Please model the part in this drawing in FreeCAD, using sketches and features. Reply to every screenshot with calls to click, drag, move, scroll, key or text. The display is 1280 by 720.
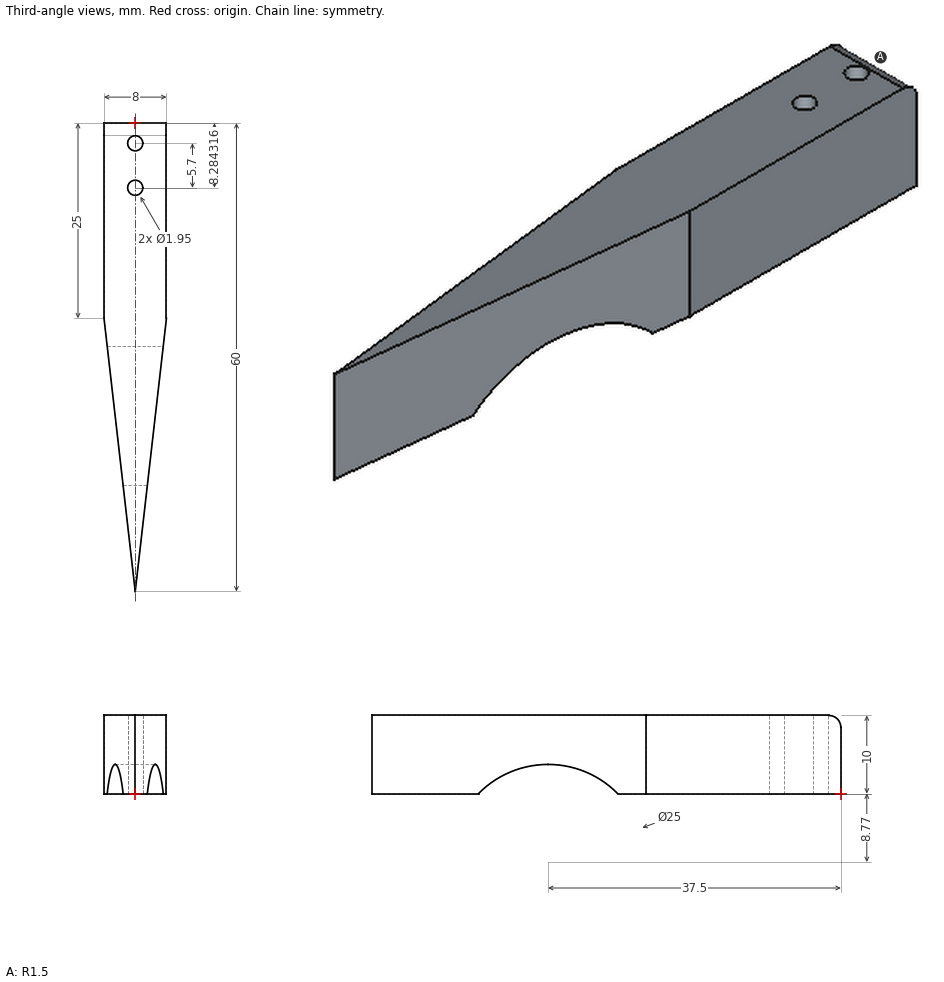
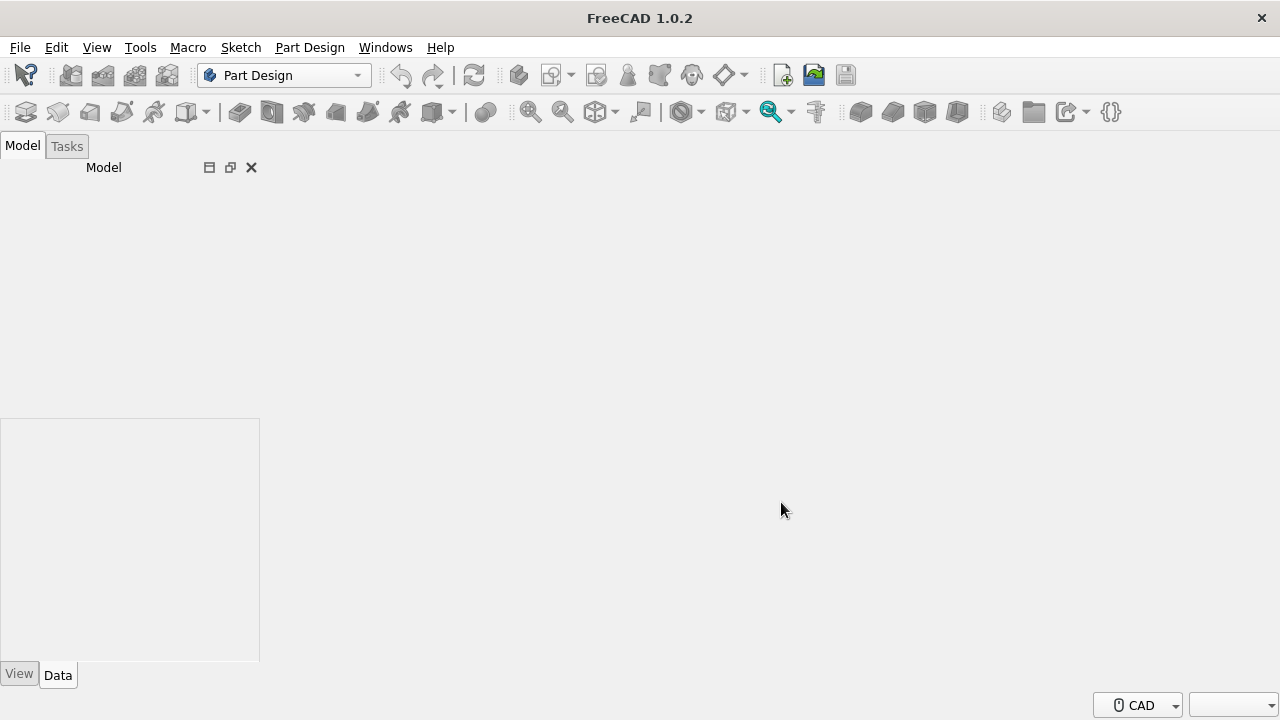
key(ctrl+n)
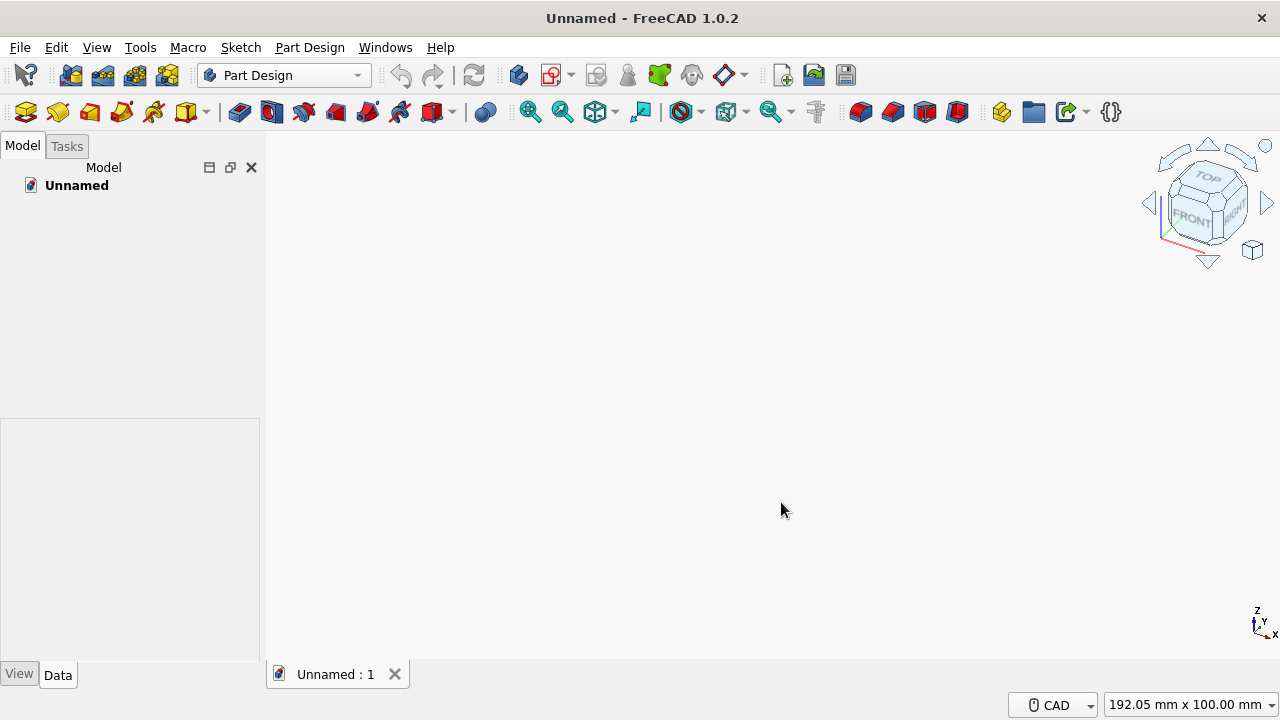
click(552, 76)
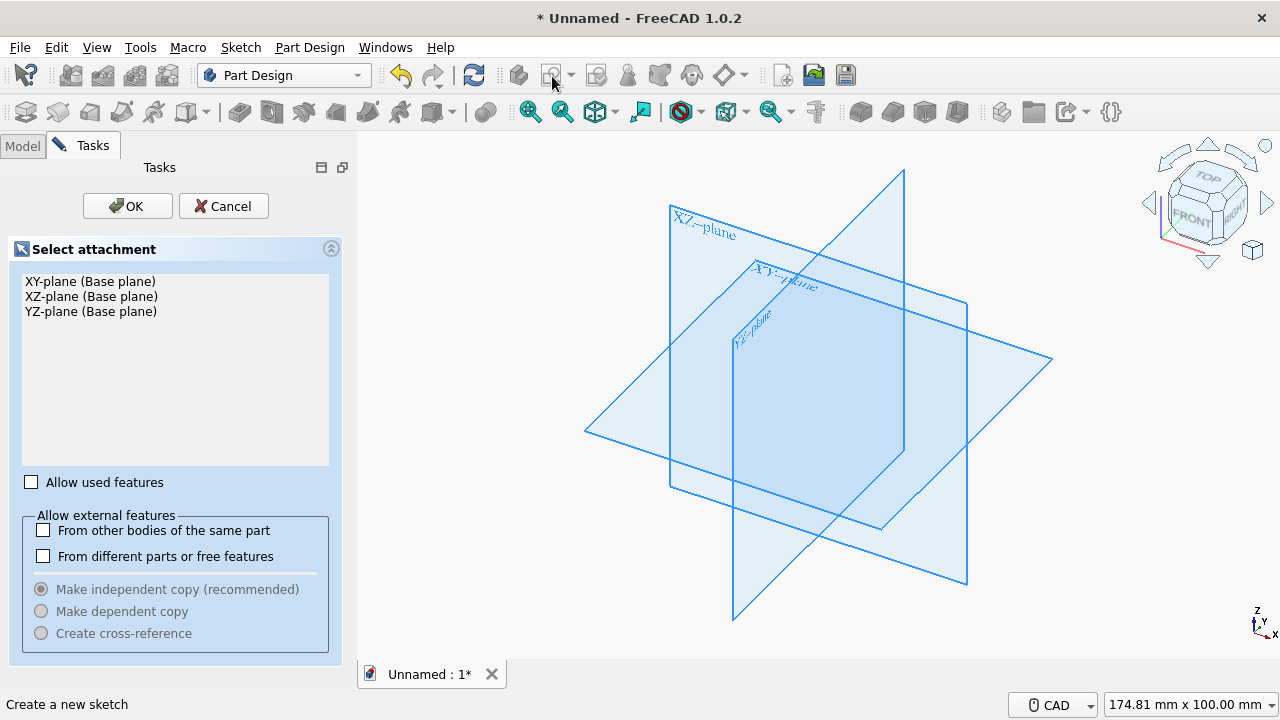
click(82, 282)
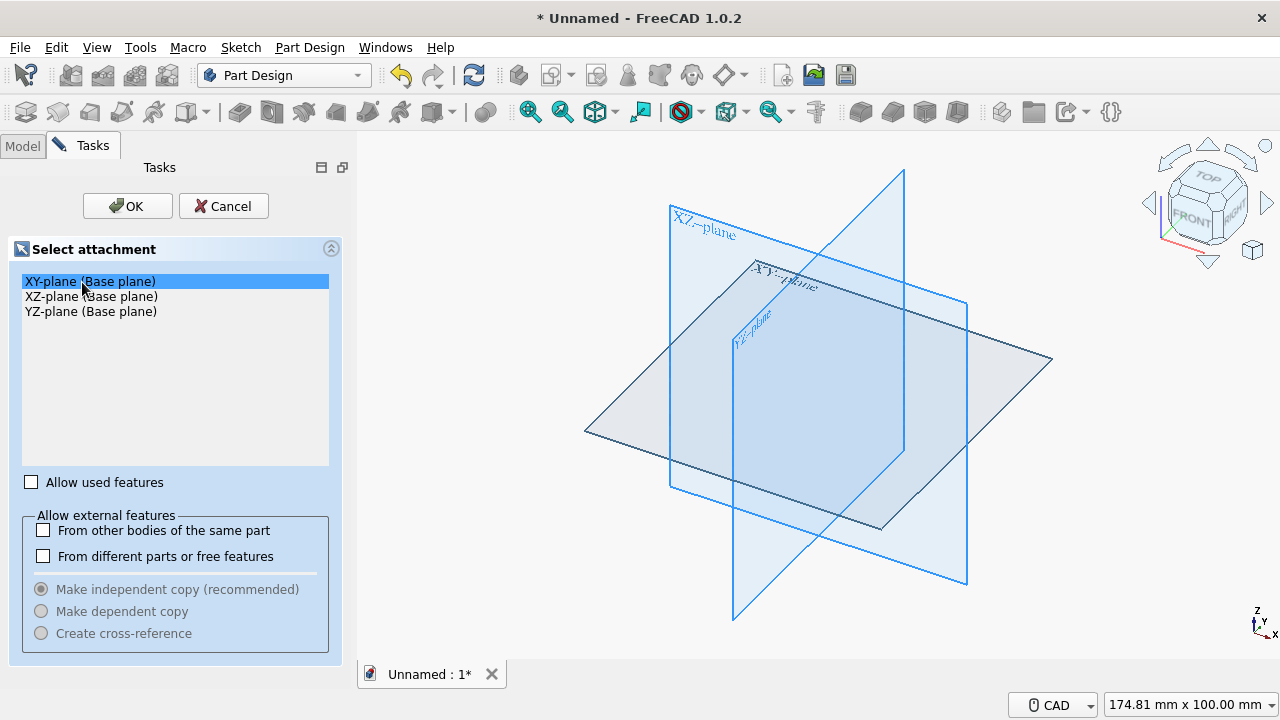
click(128, 206)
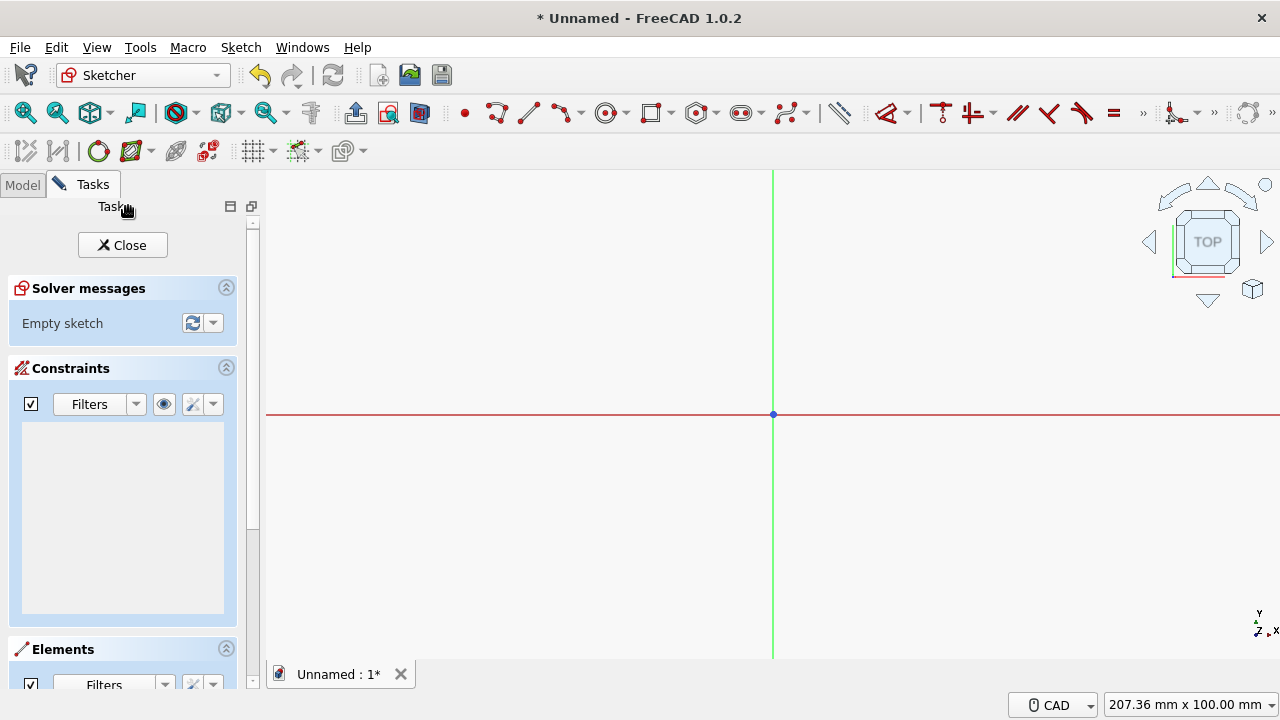
scroll(565, 198, down, 2)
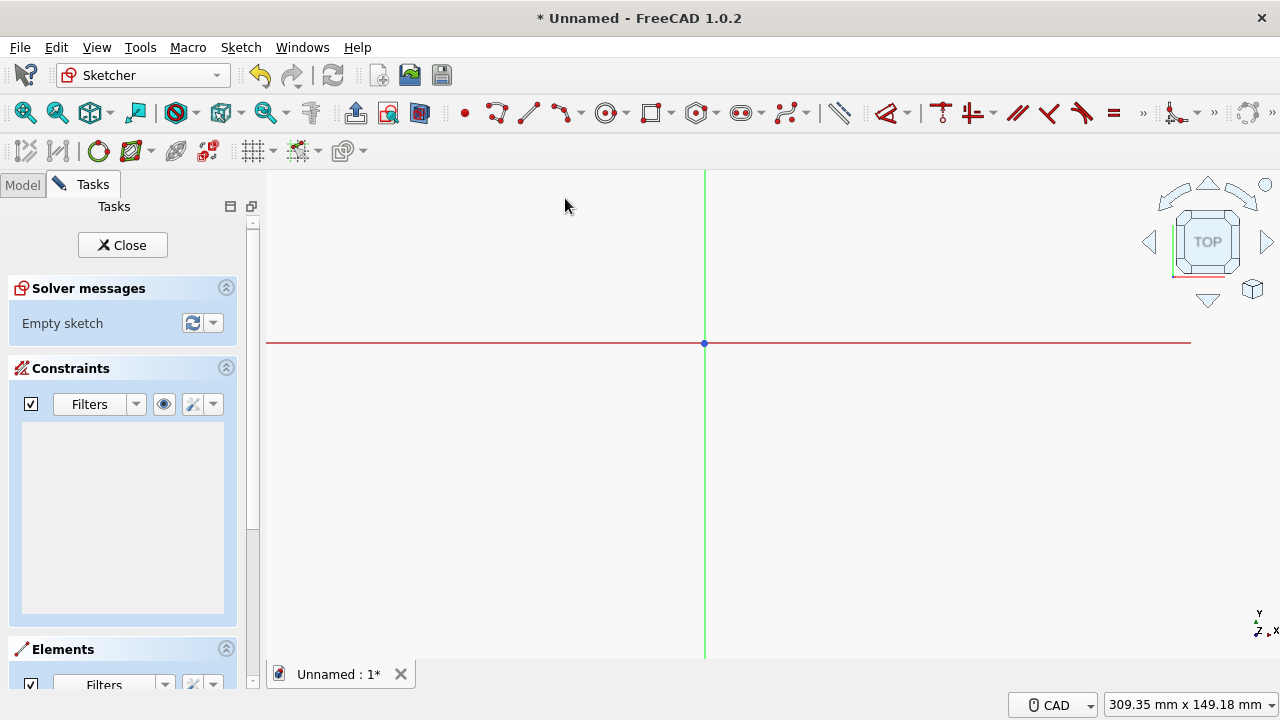
scroll(705, 496, up, 2)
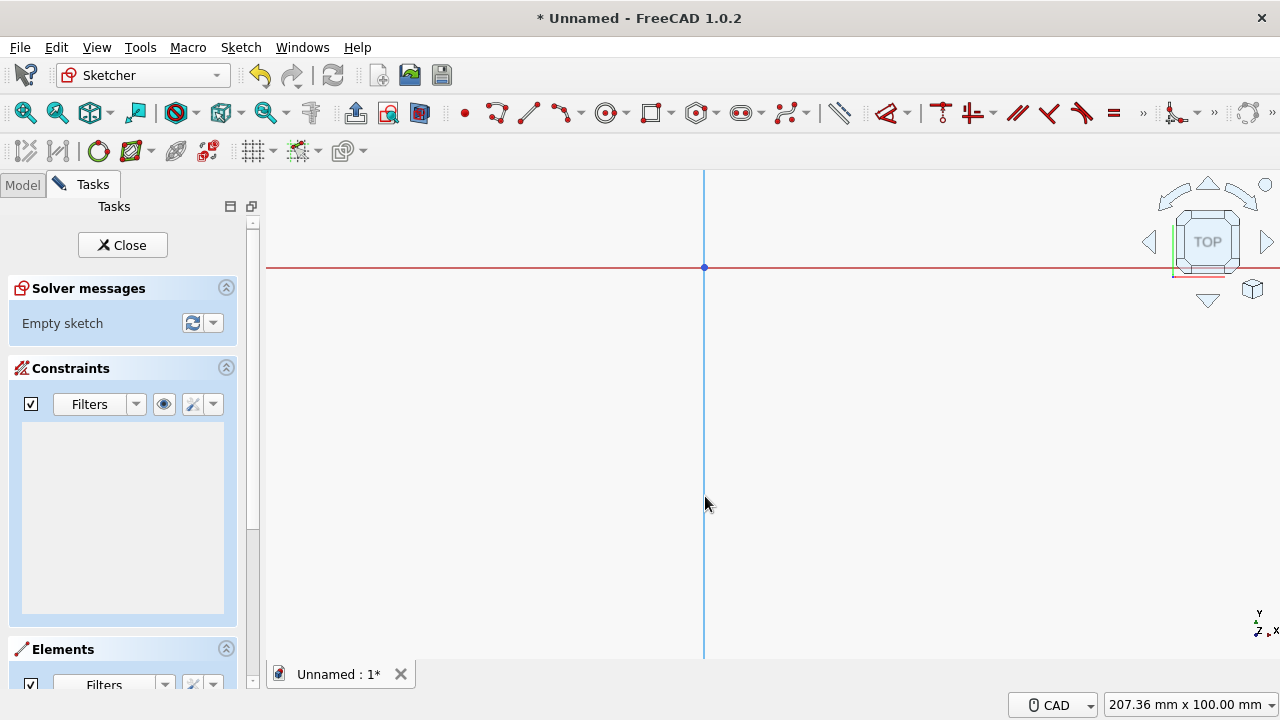
click(498, 114)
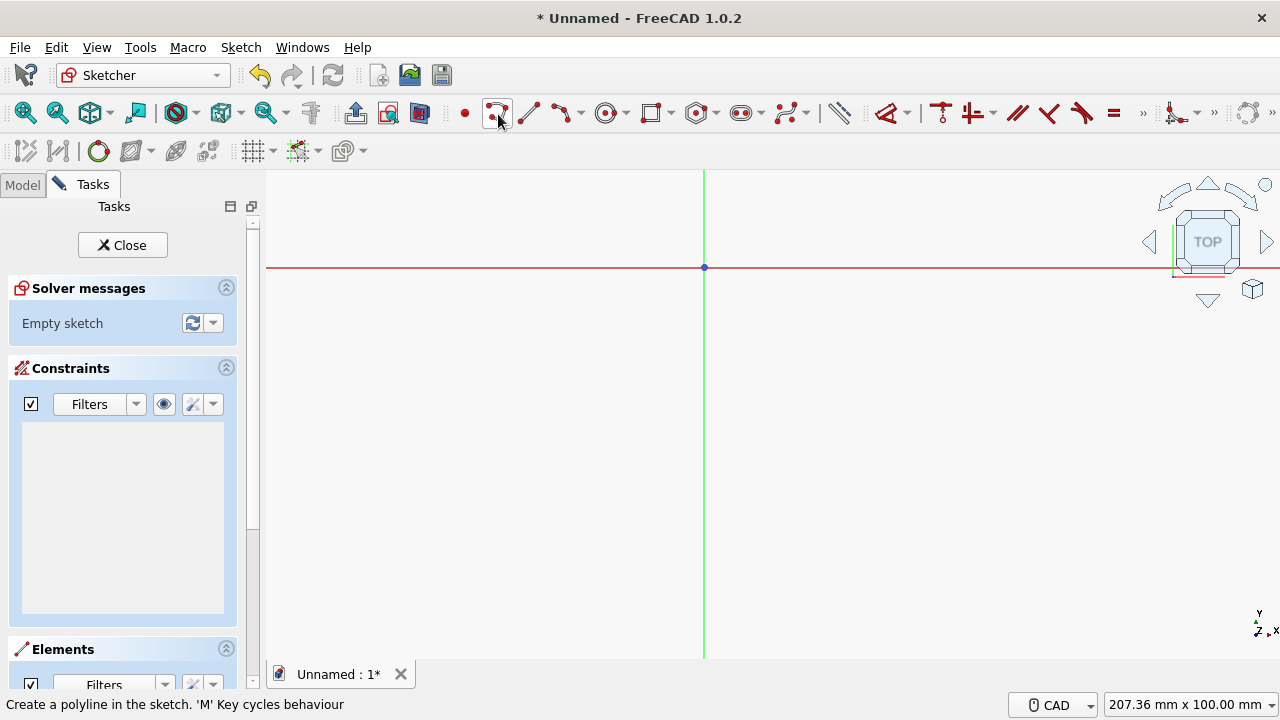
click(724, 268)
click(685, 277)
click(685, 390)
click(704, 561)
click(724, 390)
click(724, 268)
key(Escape)
key(Escape)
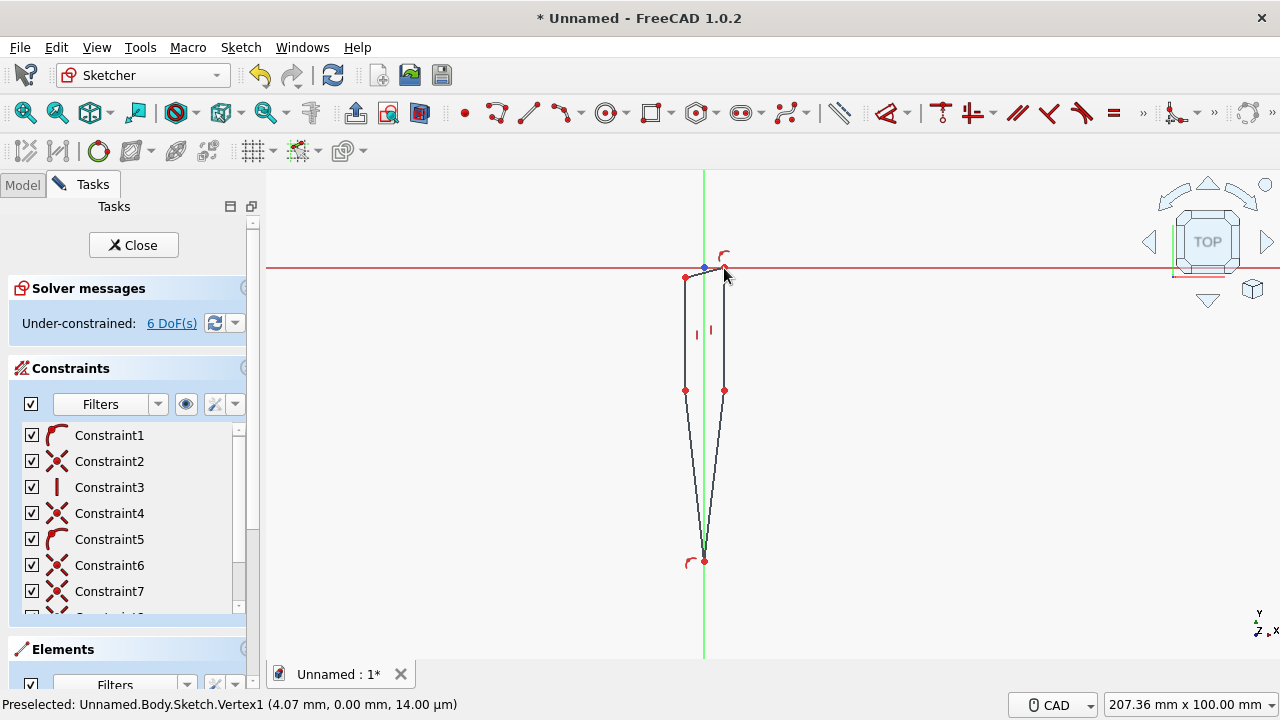
scroll(712, 271, up, 3)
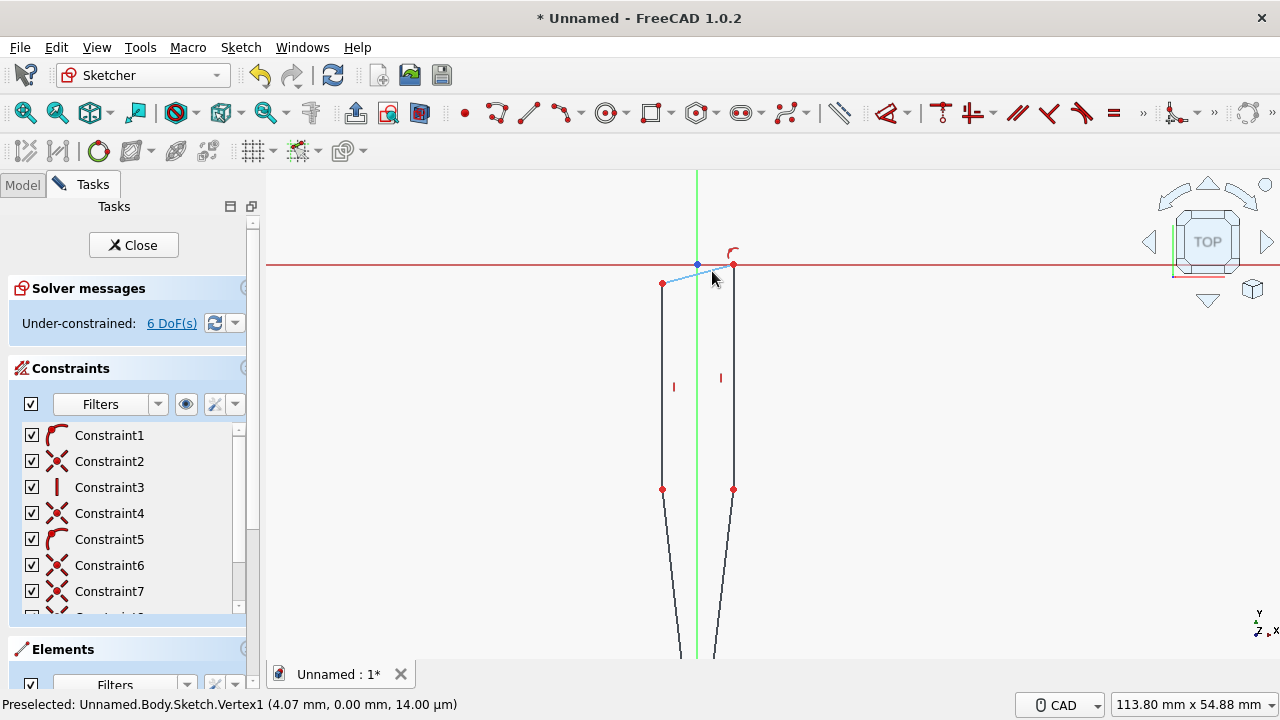
click(712, 270)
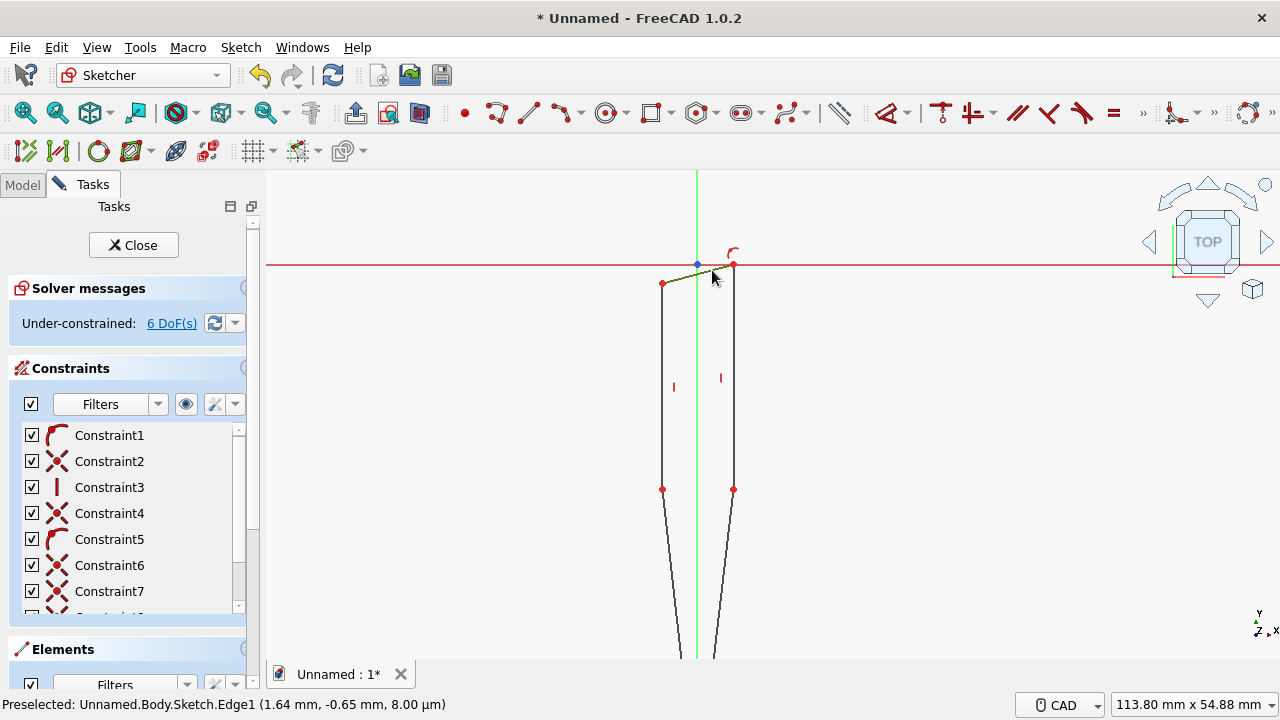
key(h)